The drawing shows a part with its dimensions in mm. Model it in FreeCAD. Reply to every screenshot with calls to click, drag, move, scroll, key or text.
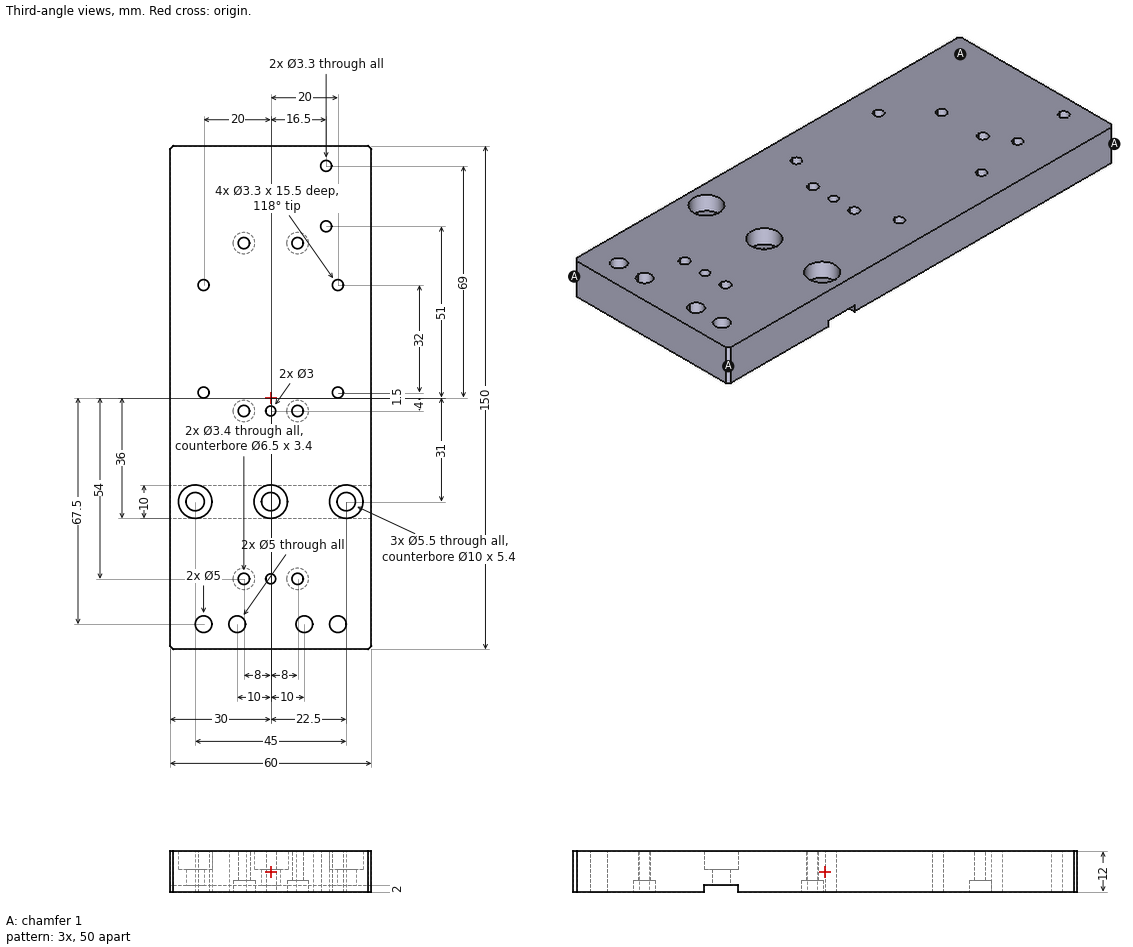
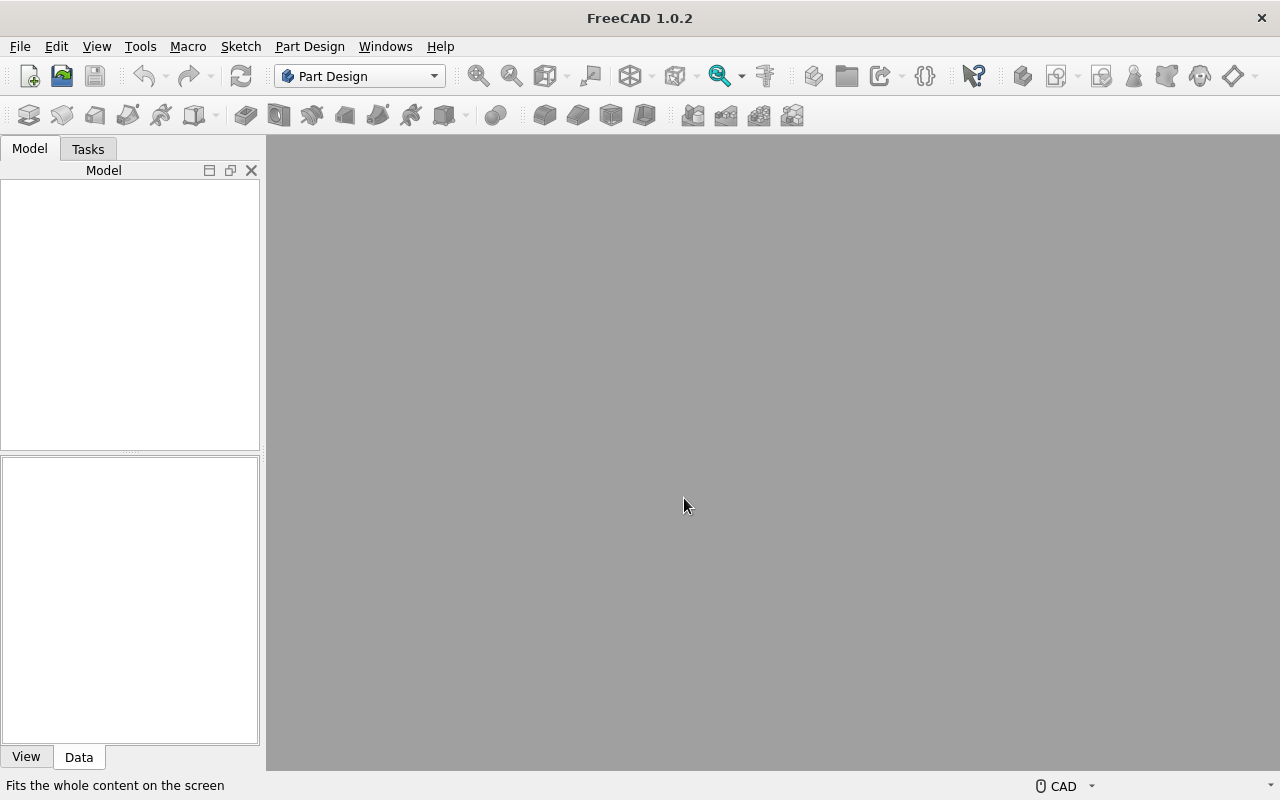
click(29, 76)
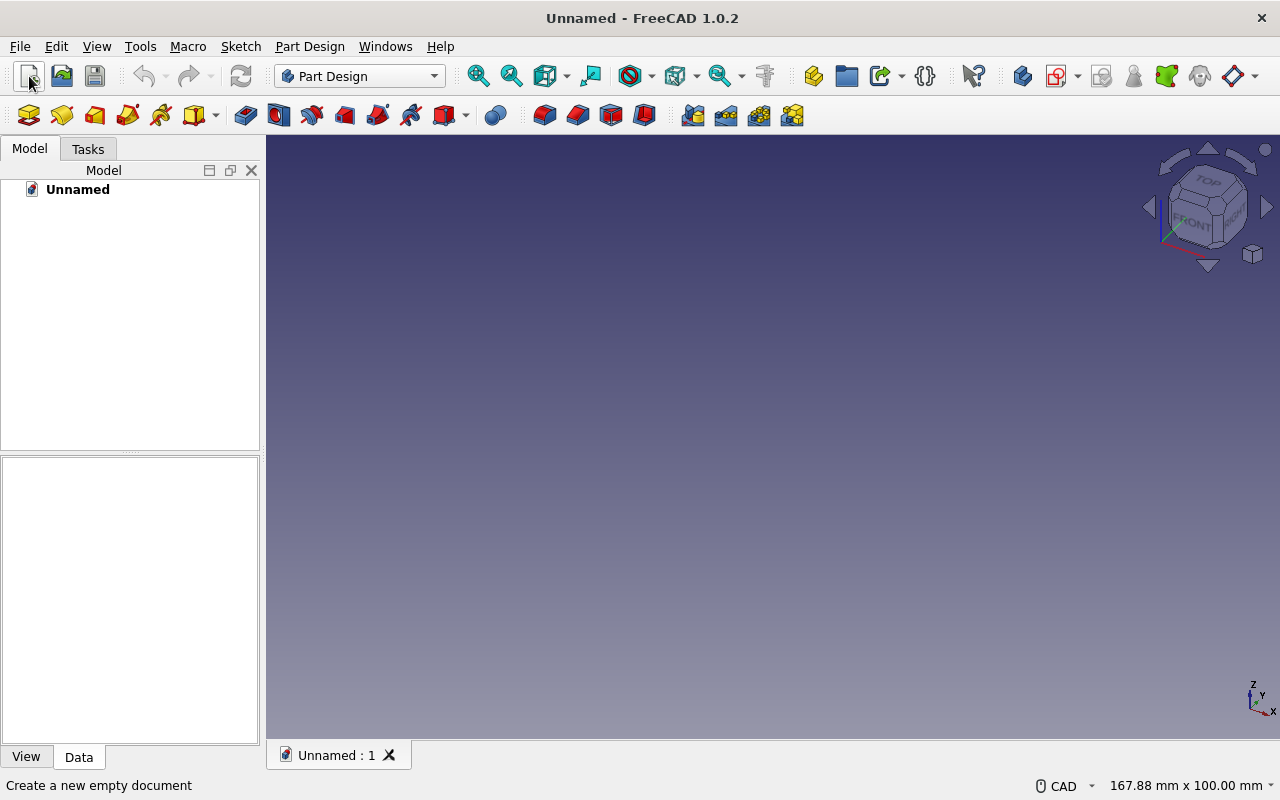
click(1056, 76)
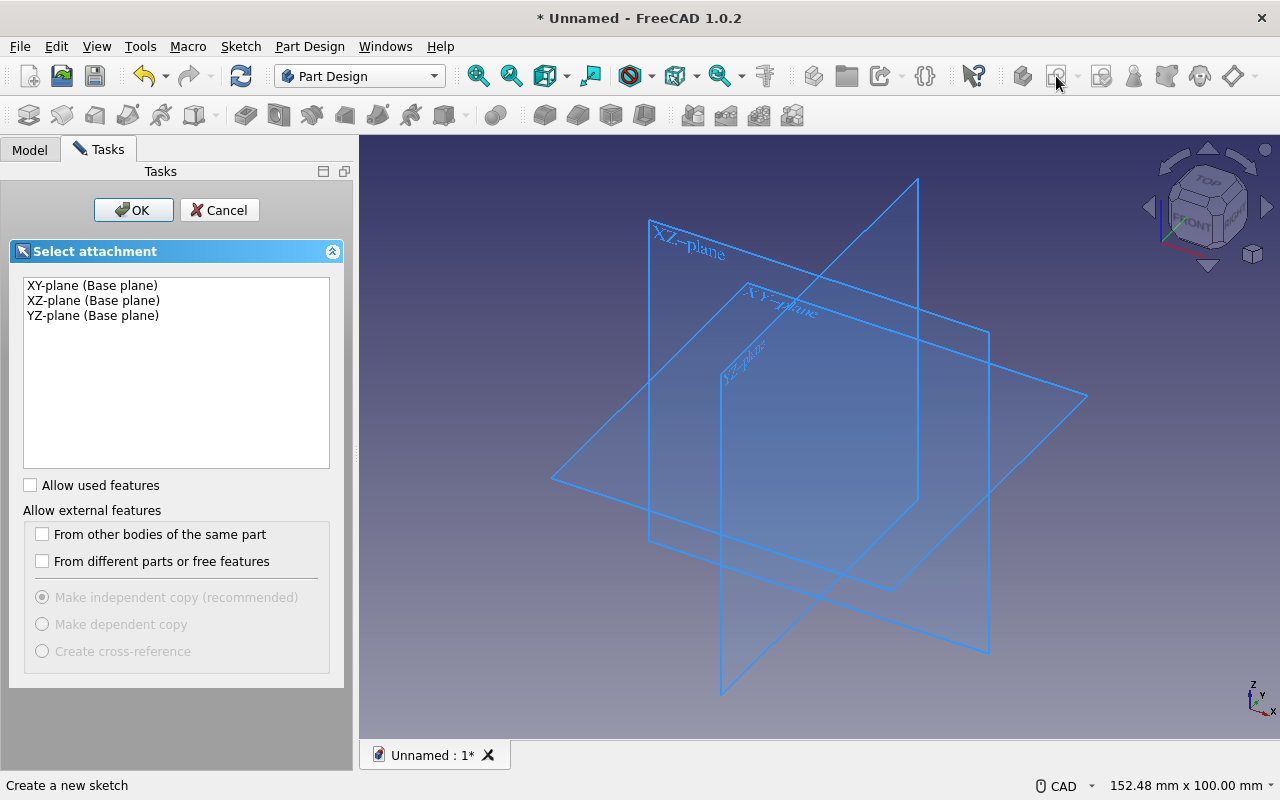
click(84, 286)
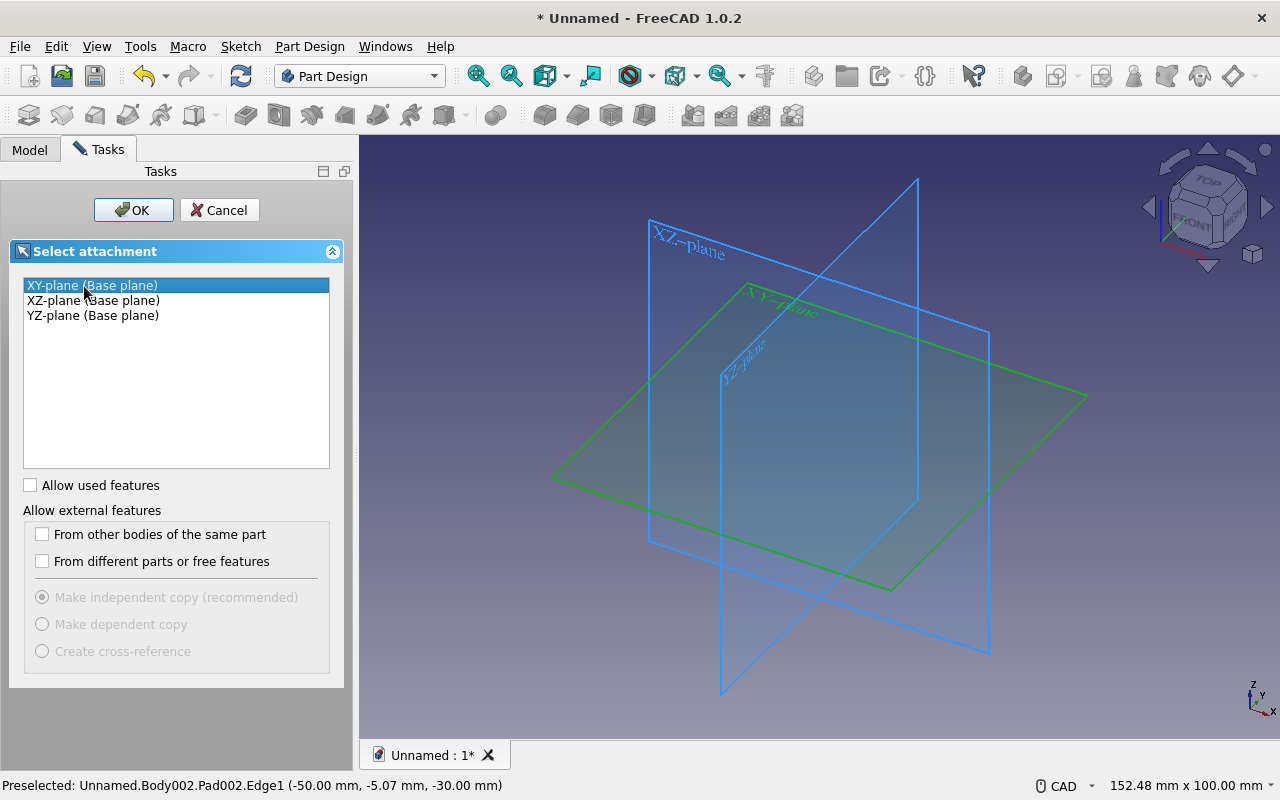
click(134, 210)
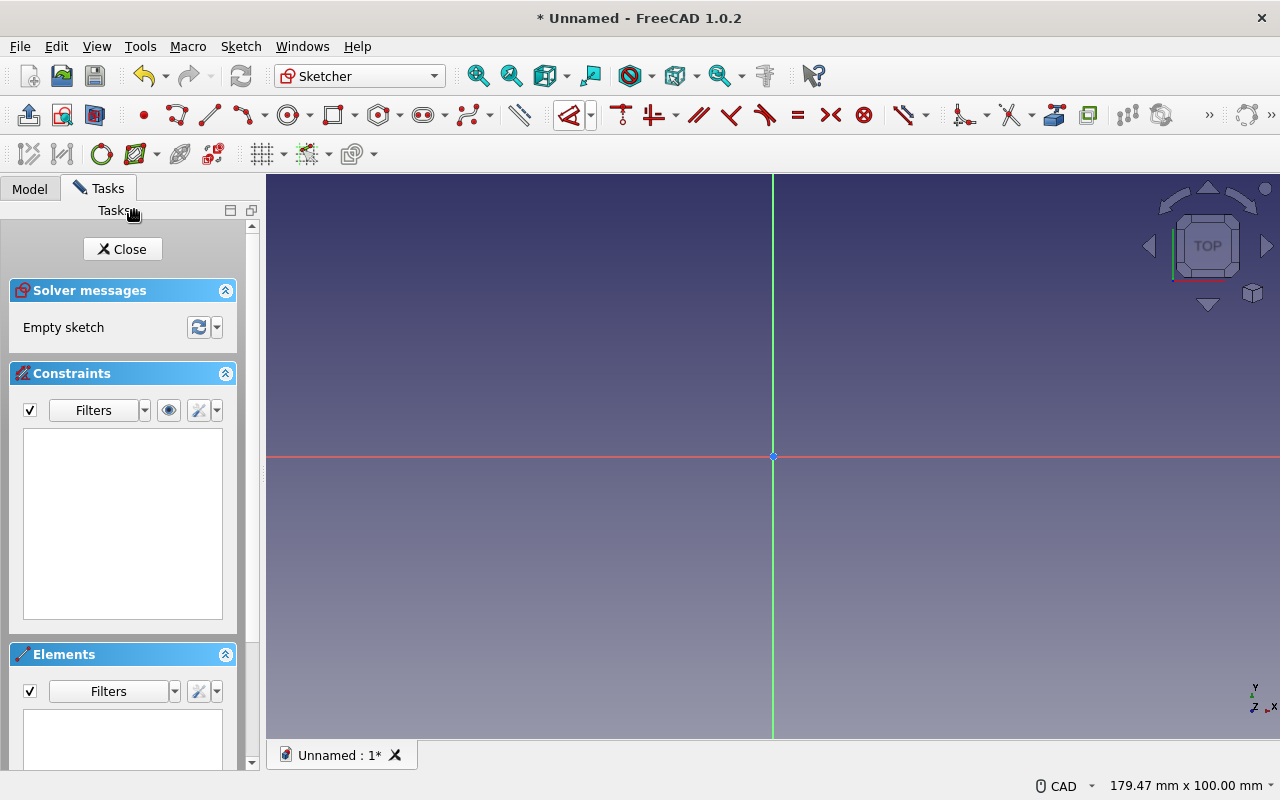
scroll(649, 456, down, 4)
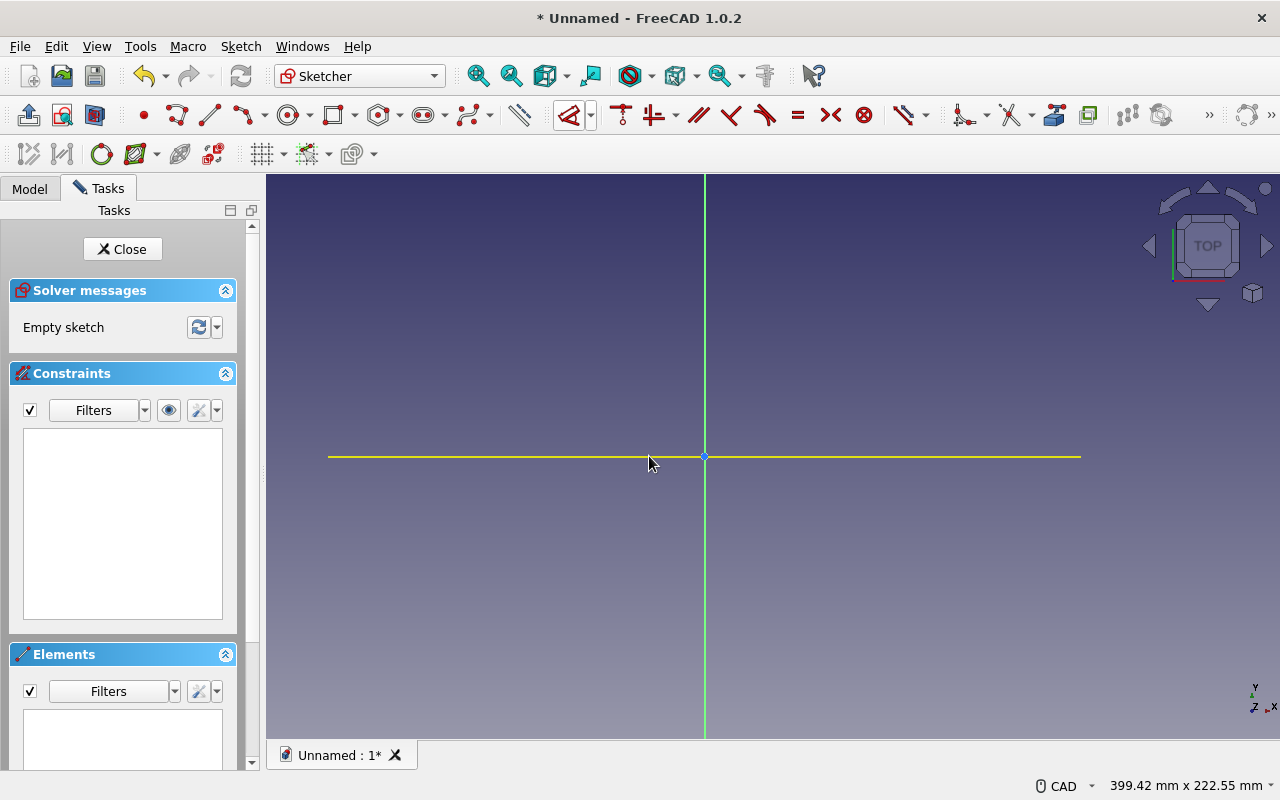
key(g)
key(v)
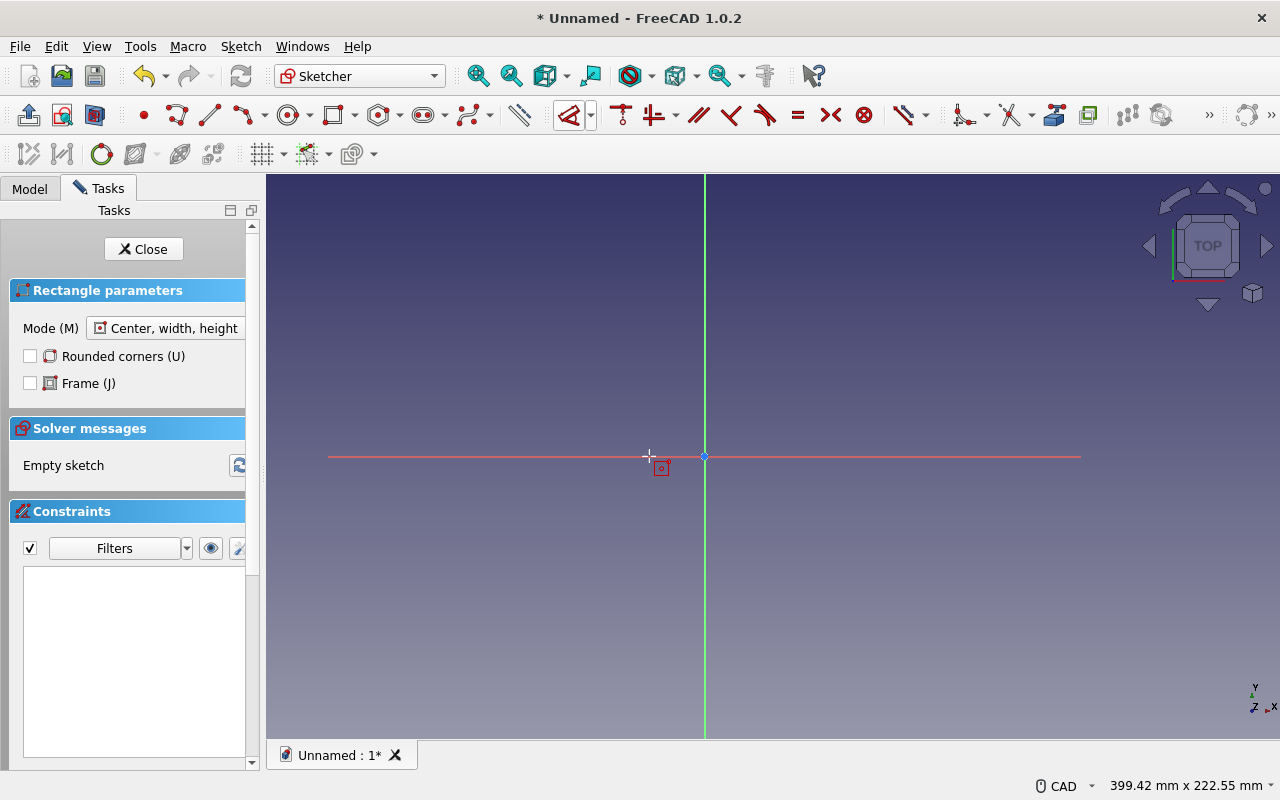
click(705, 456)
click(781, 266)
key(Escape)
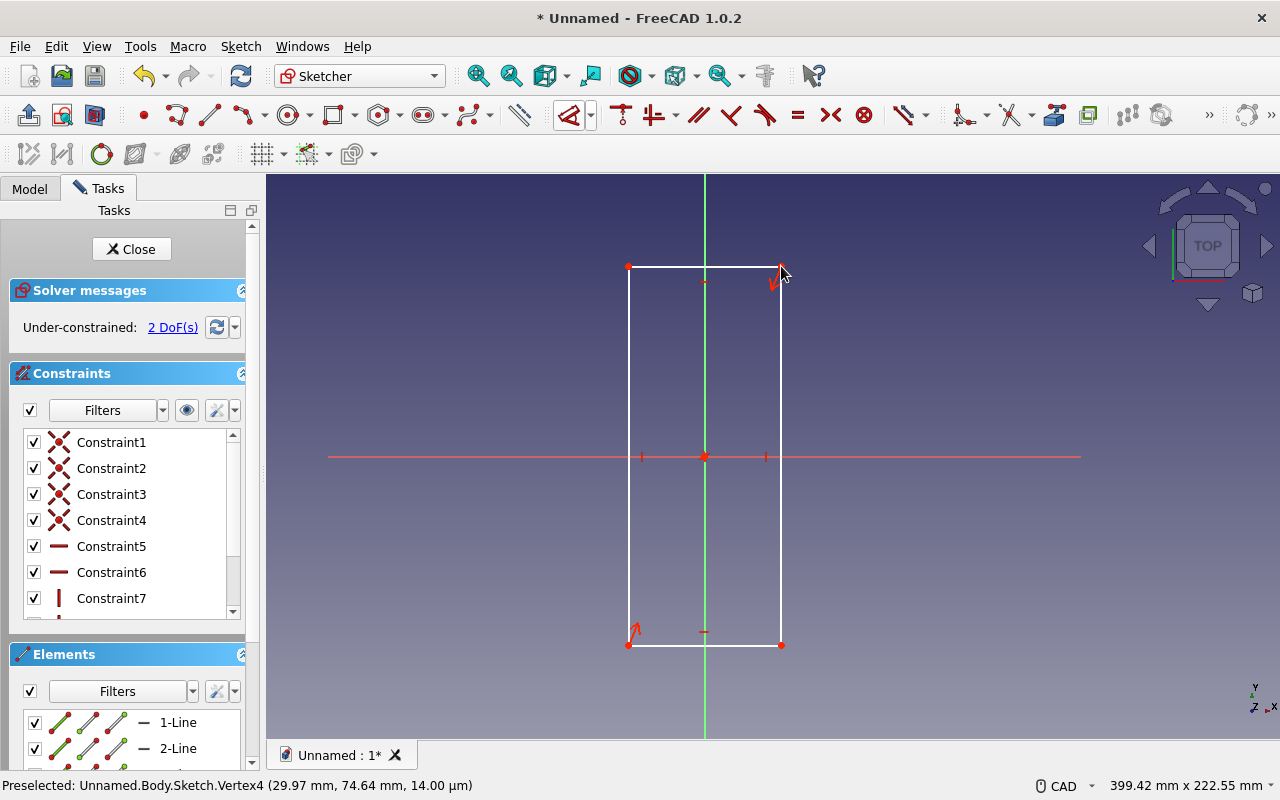
click(568, 116)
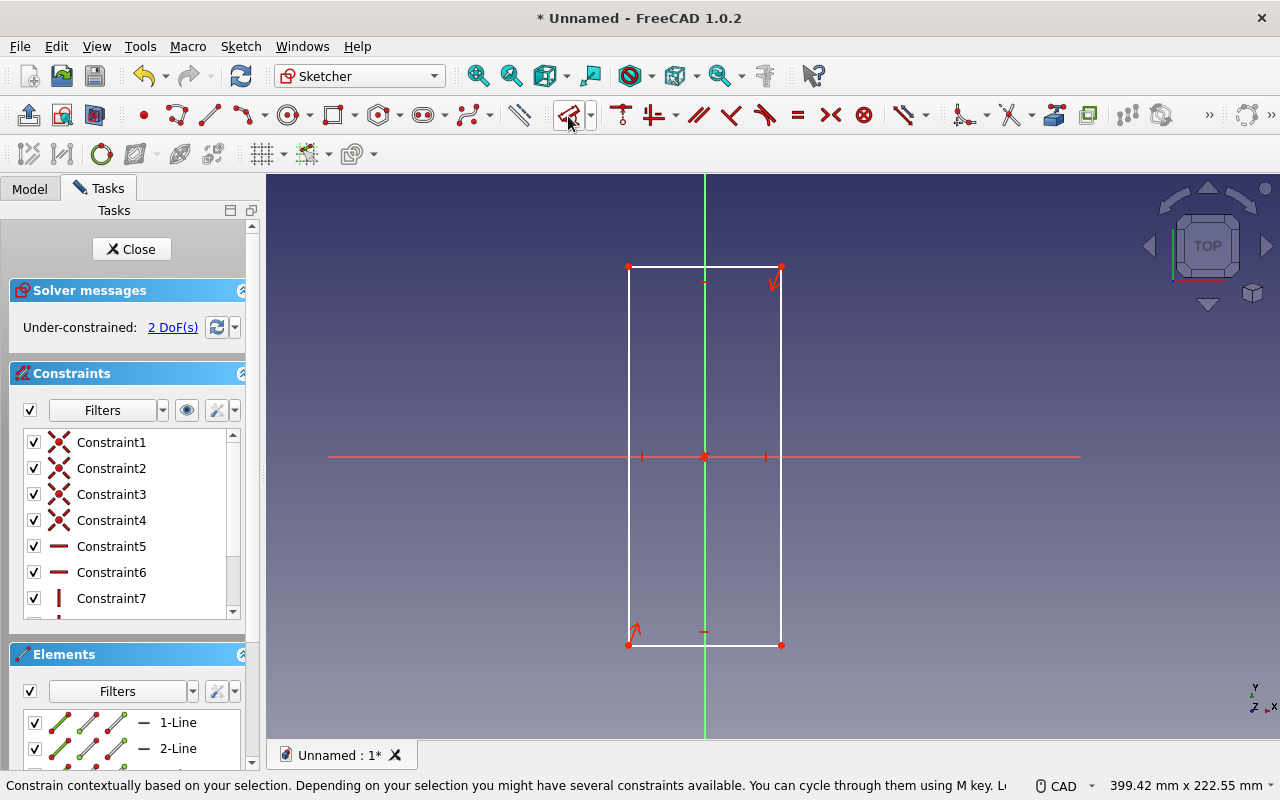
click(674, 646)
click(670, 680)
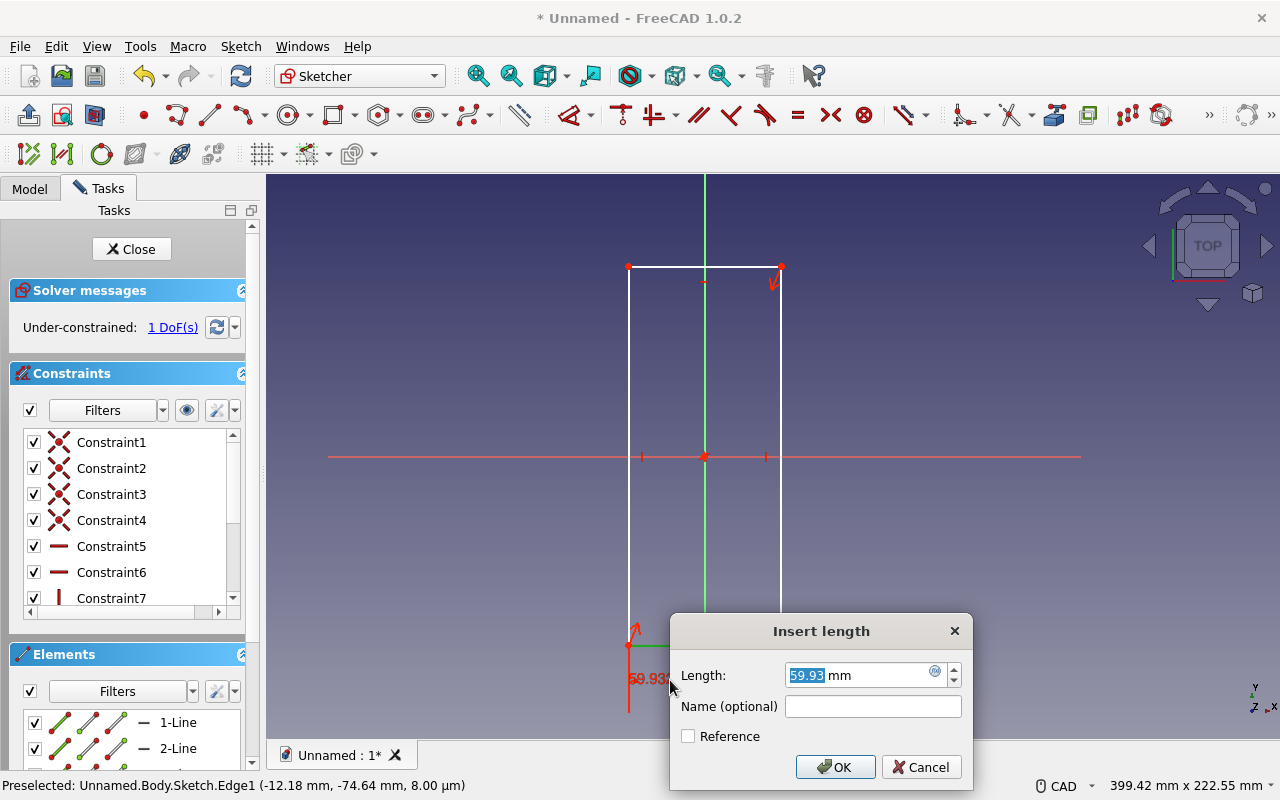
text(60)
key(Return)